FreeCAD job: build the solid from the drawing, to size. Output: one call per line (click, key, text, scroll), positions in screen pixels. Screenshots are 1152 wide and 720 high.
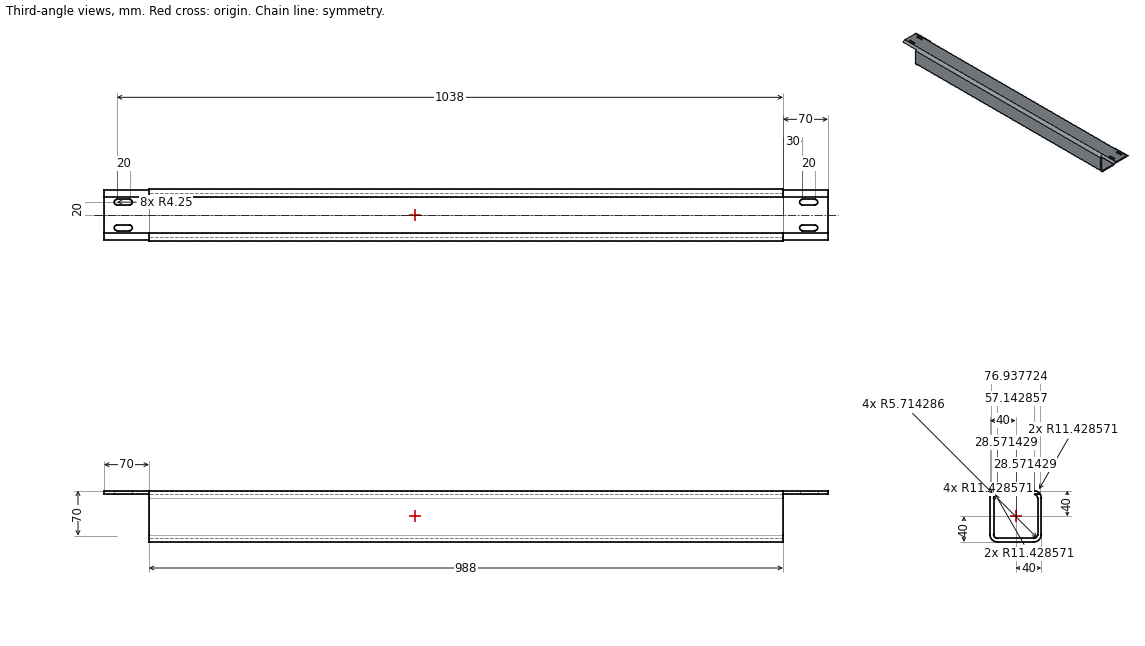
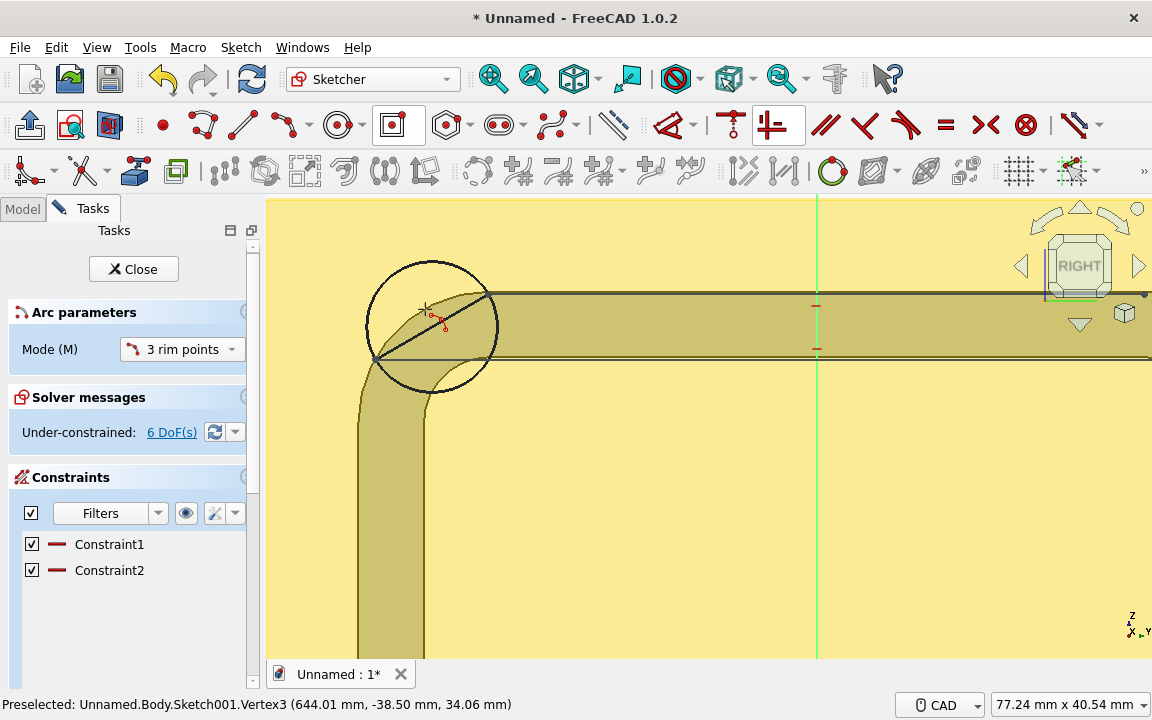
click(424, 309)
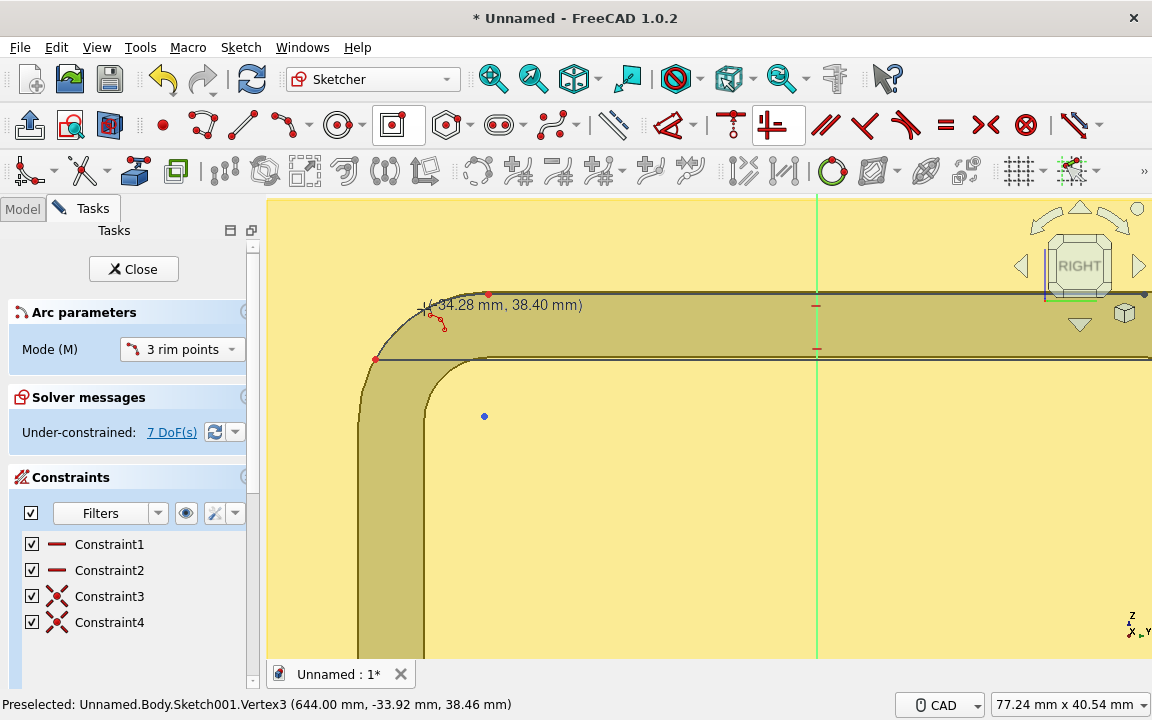
scroll(425, 311, down, 3)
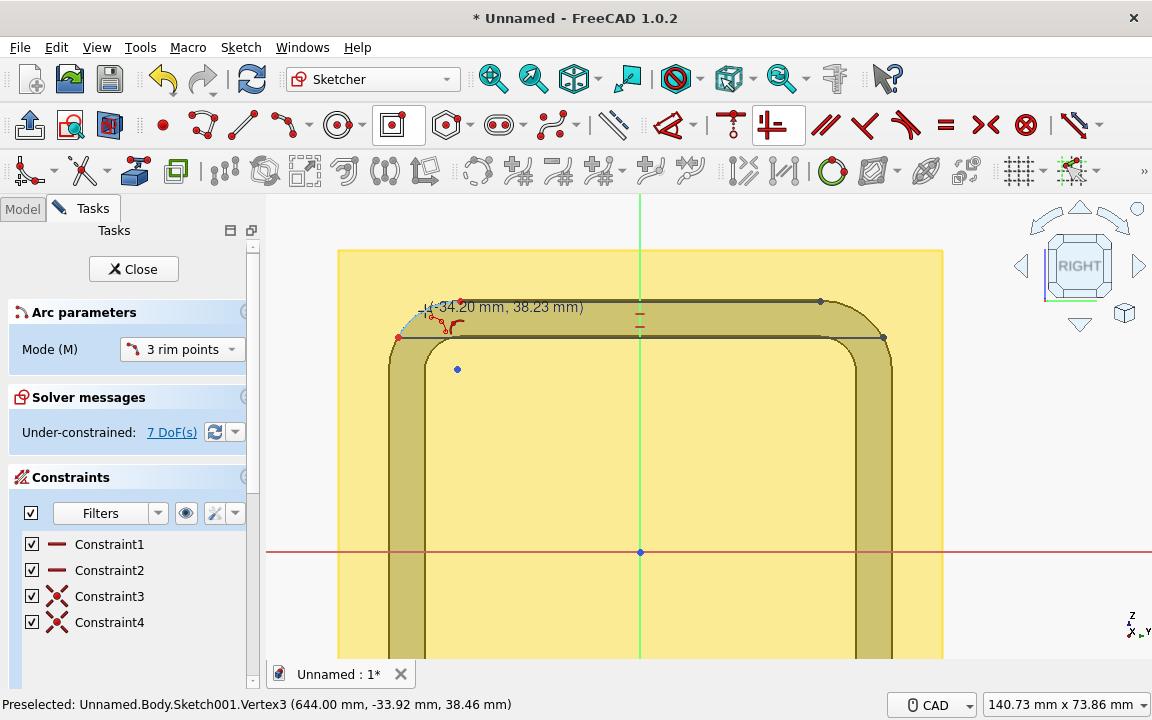
click(883, 338)
click(820, 302)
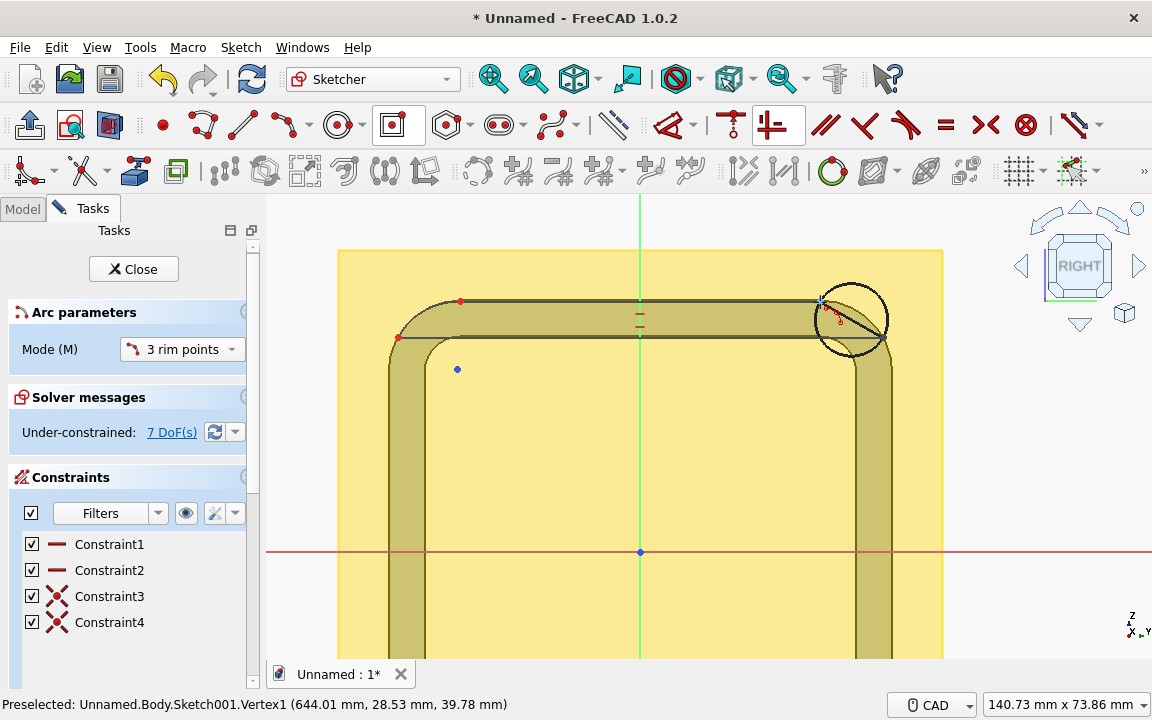
scroll(856, 310, up, 3)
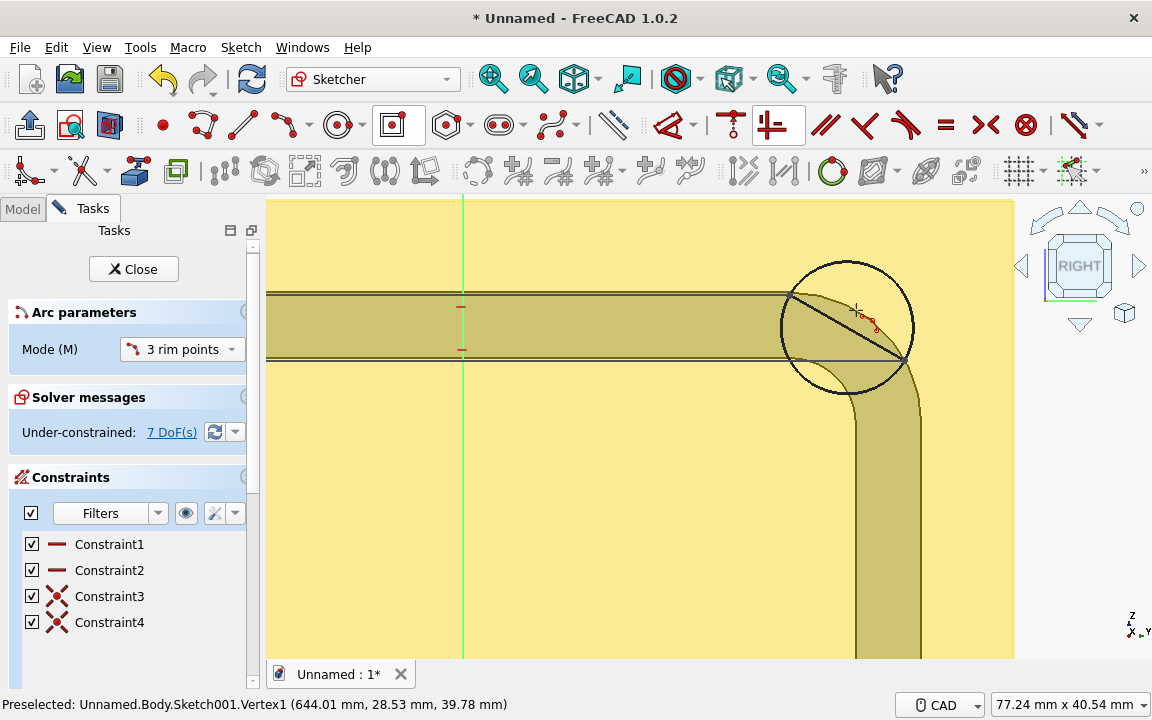
click(856, 310)
key(Escape)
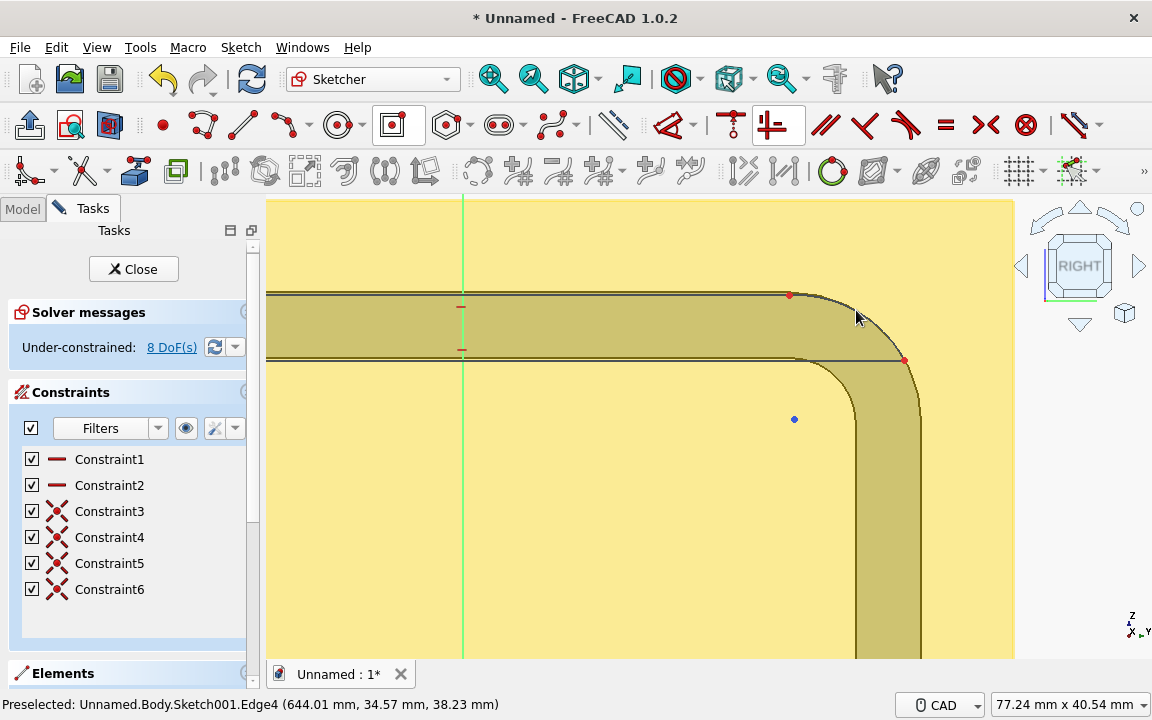
click(593, 295)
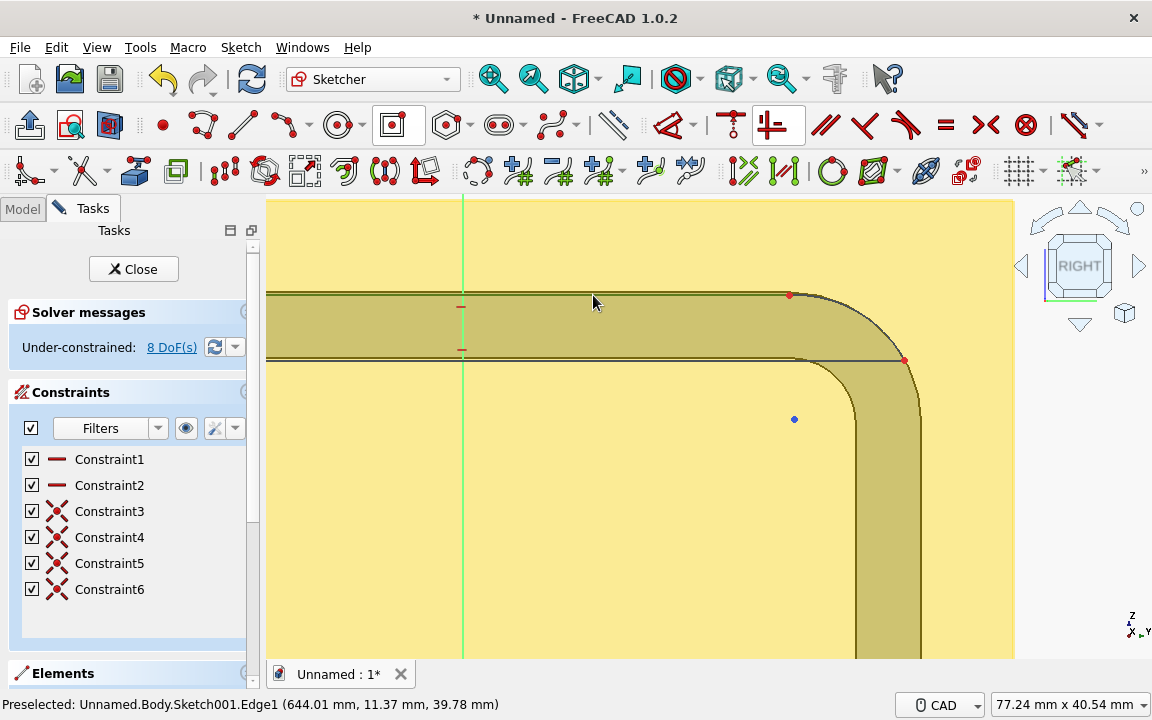
scroll(857, 310, down, 3)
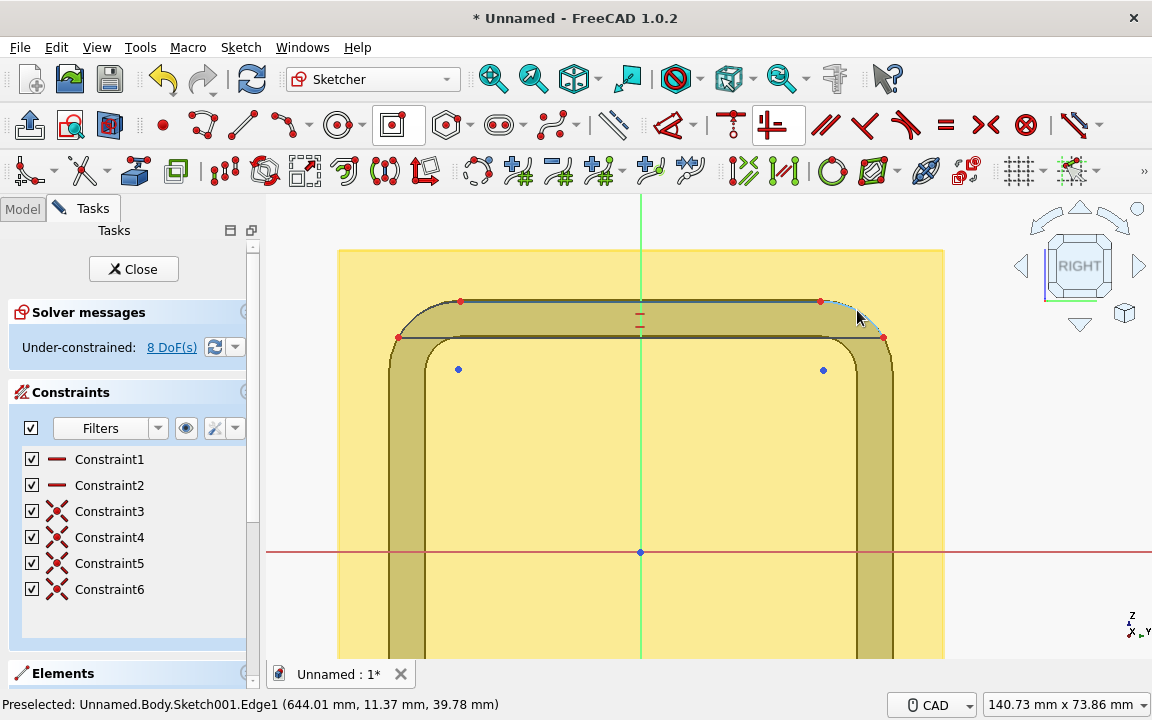
click(438, 305)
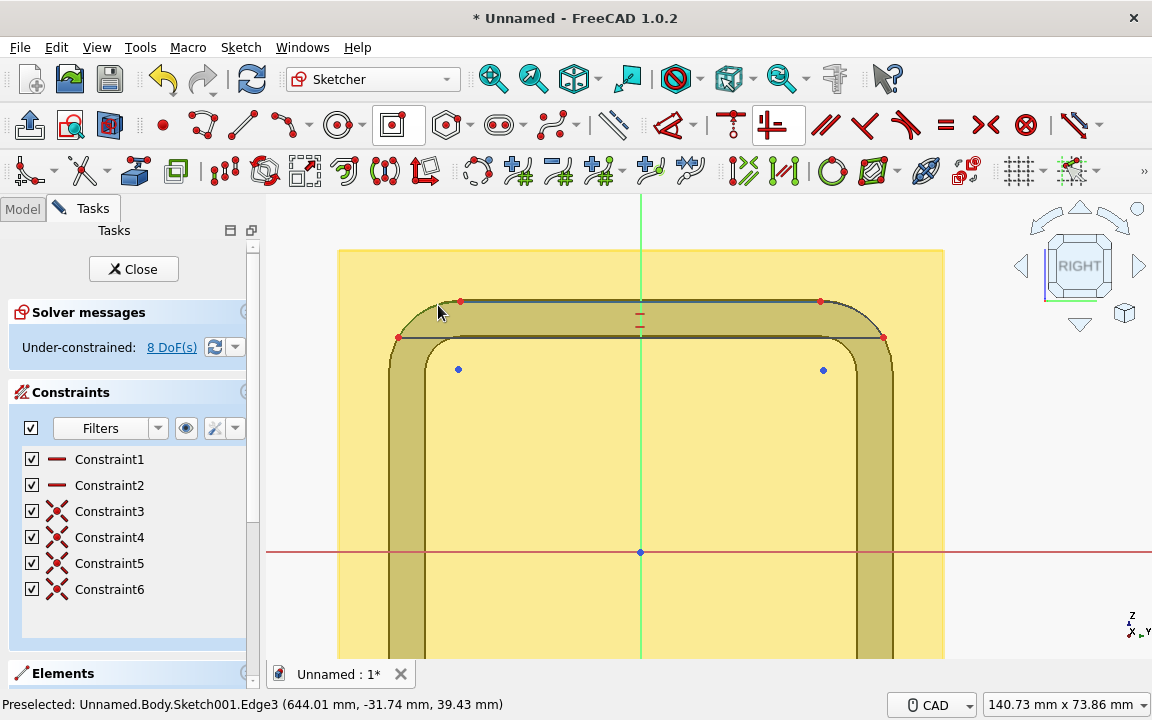
click(906, 126)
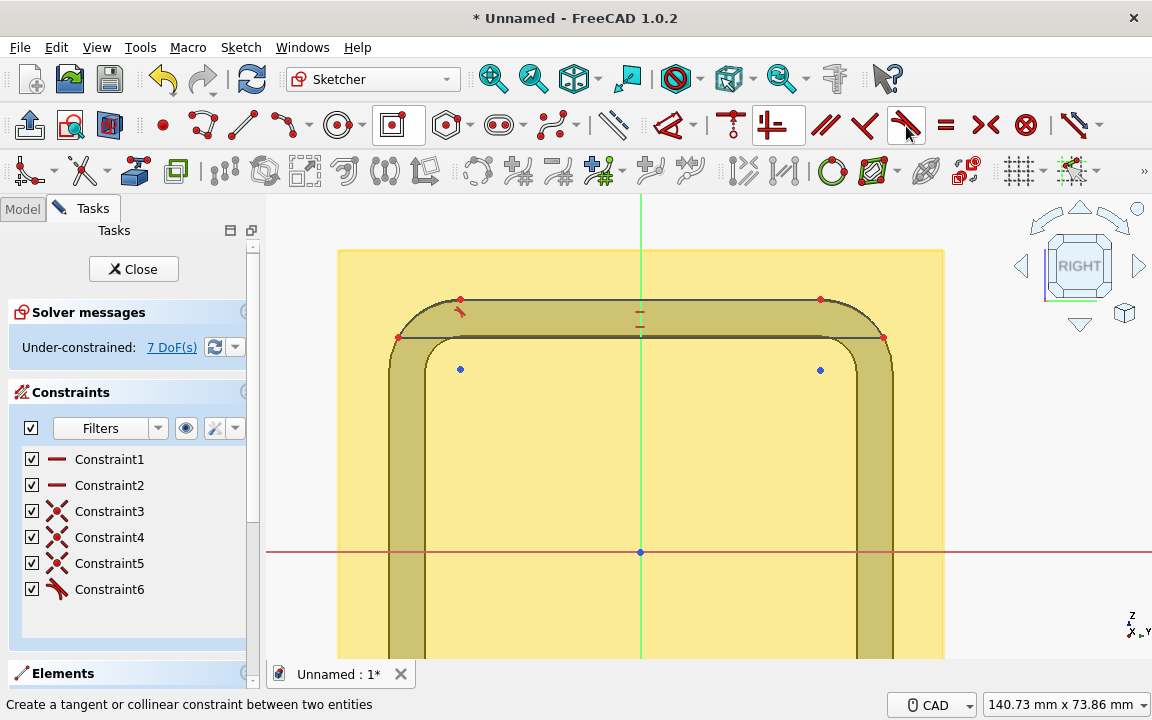
click(712, 300)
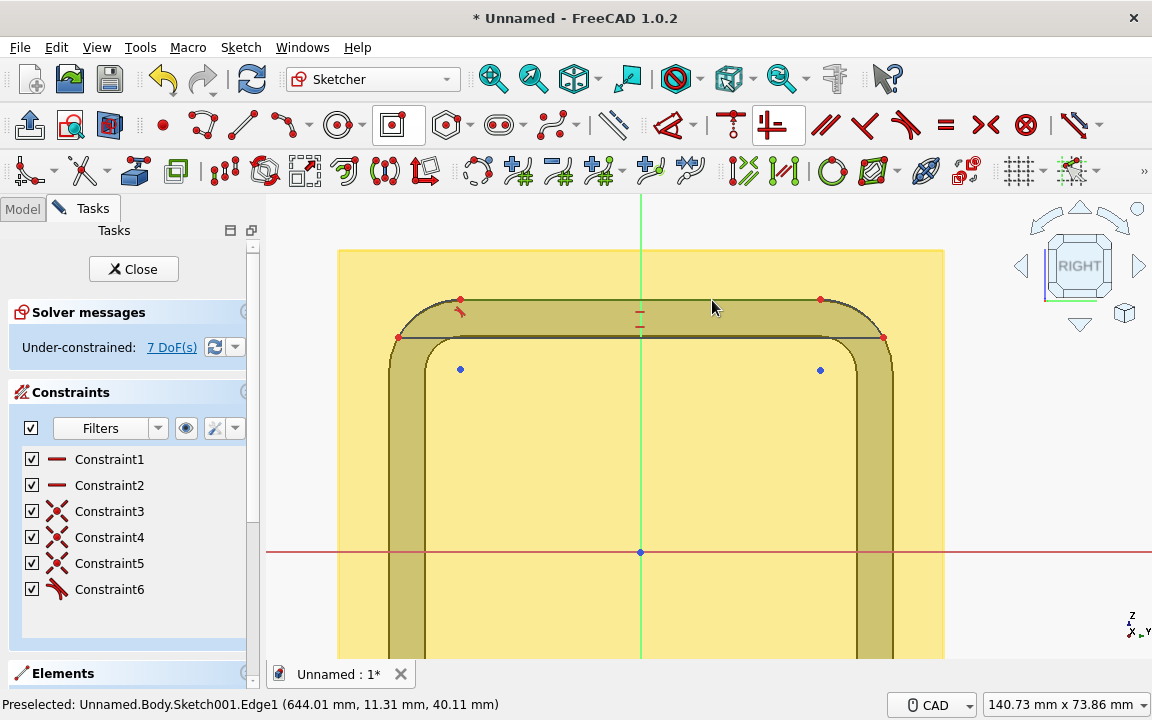
click(870, 319)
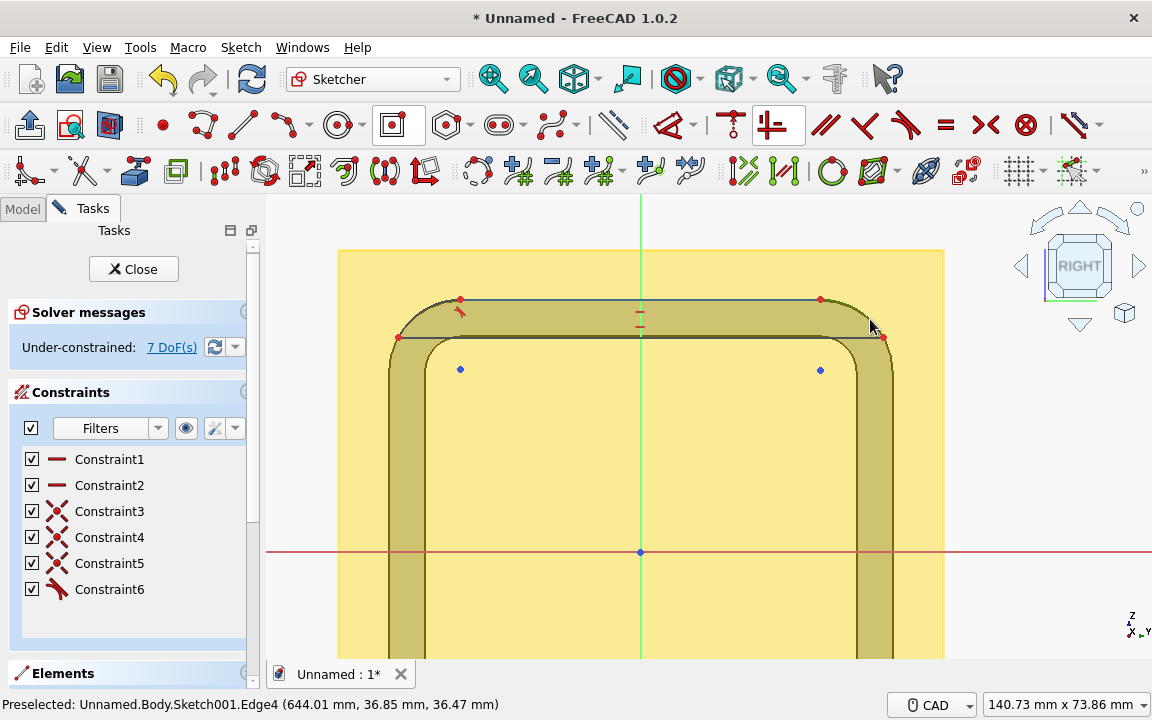
key(t)